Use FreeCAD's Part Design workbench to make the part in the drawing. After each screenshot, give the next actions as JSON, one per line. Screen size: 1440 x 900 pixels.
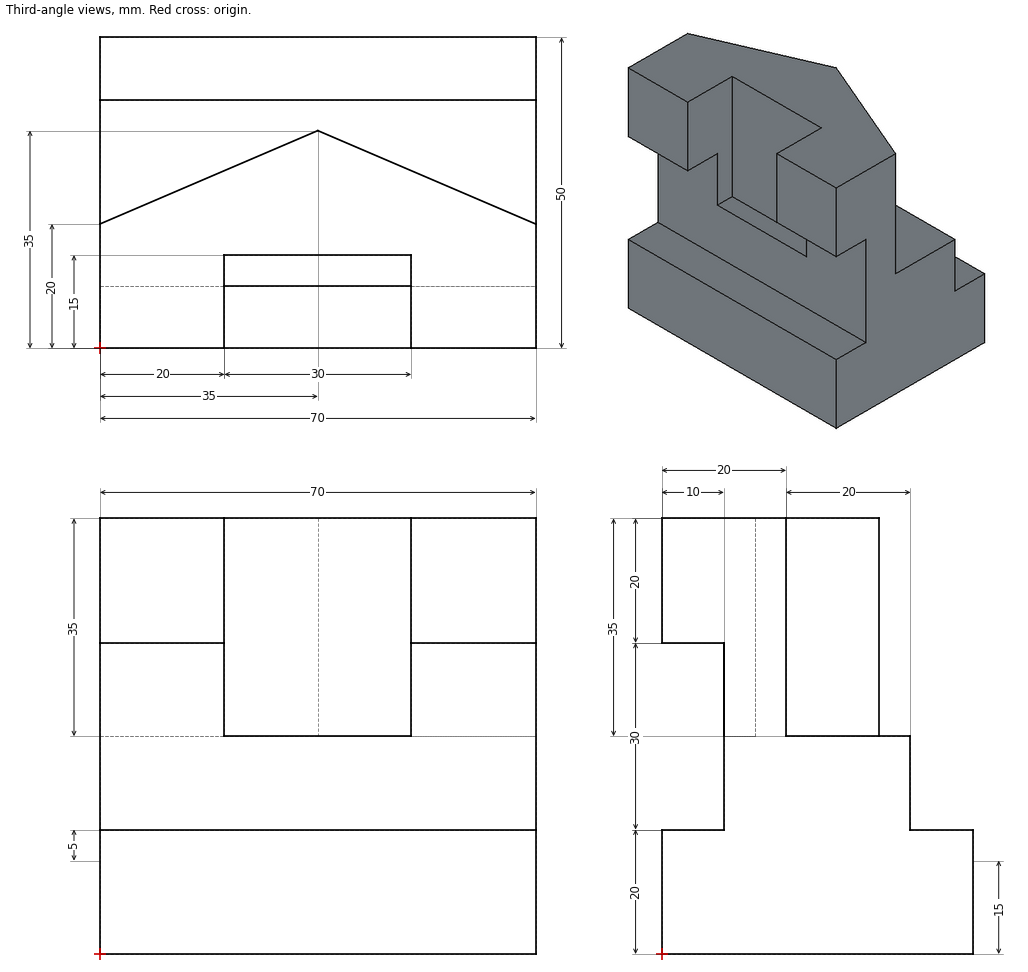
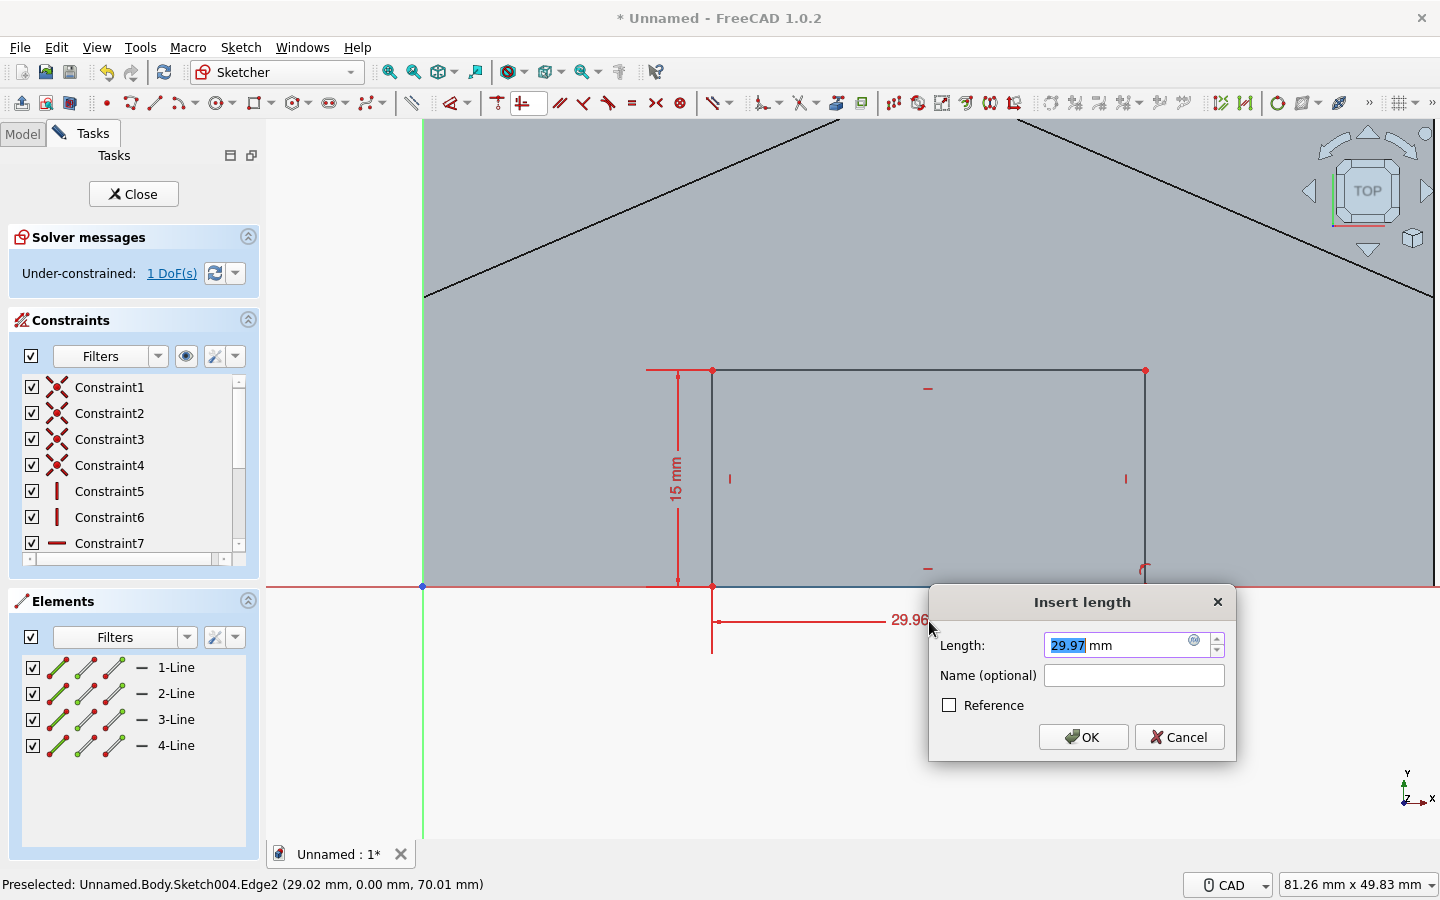
{"action": "type", "text": "30"}
{"action": "key", "text": "Return"}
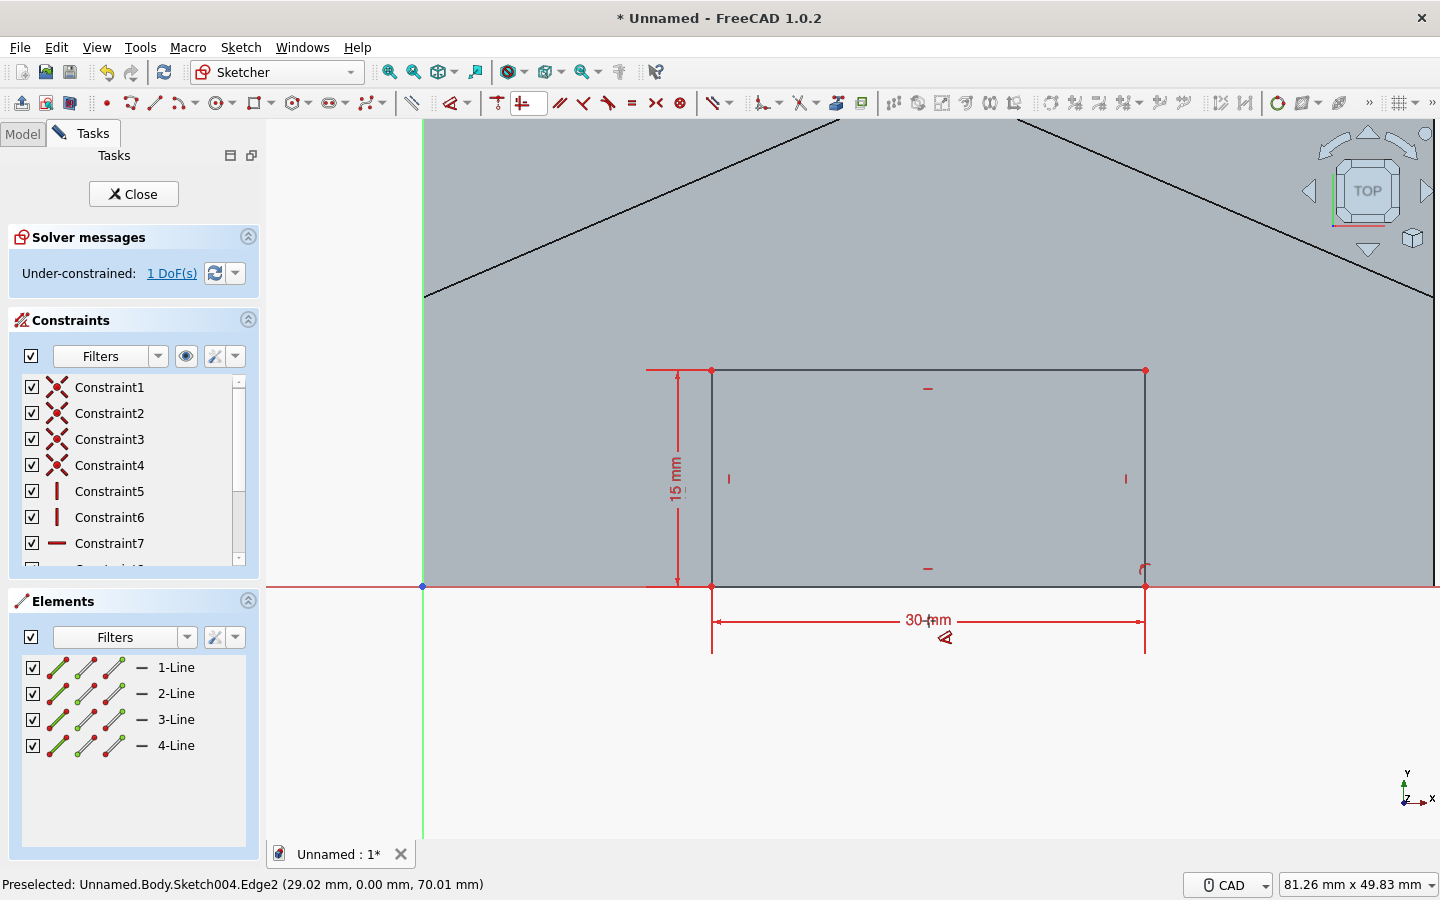
{"action": "left_click", "coordinate": [712, 370]}
{"action": "left_click", "coordinate": [567, 621]}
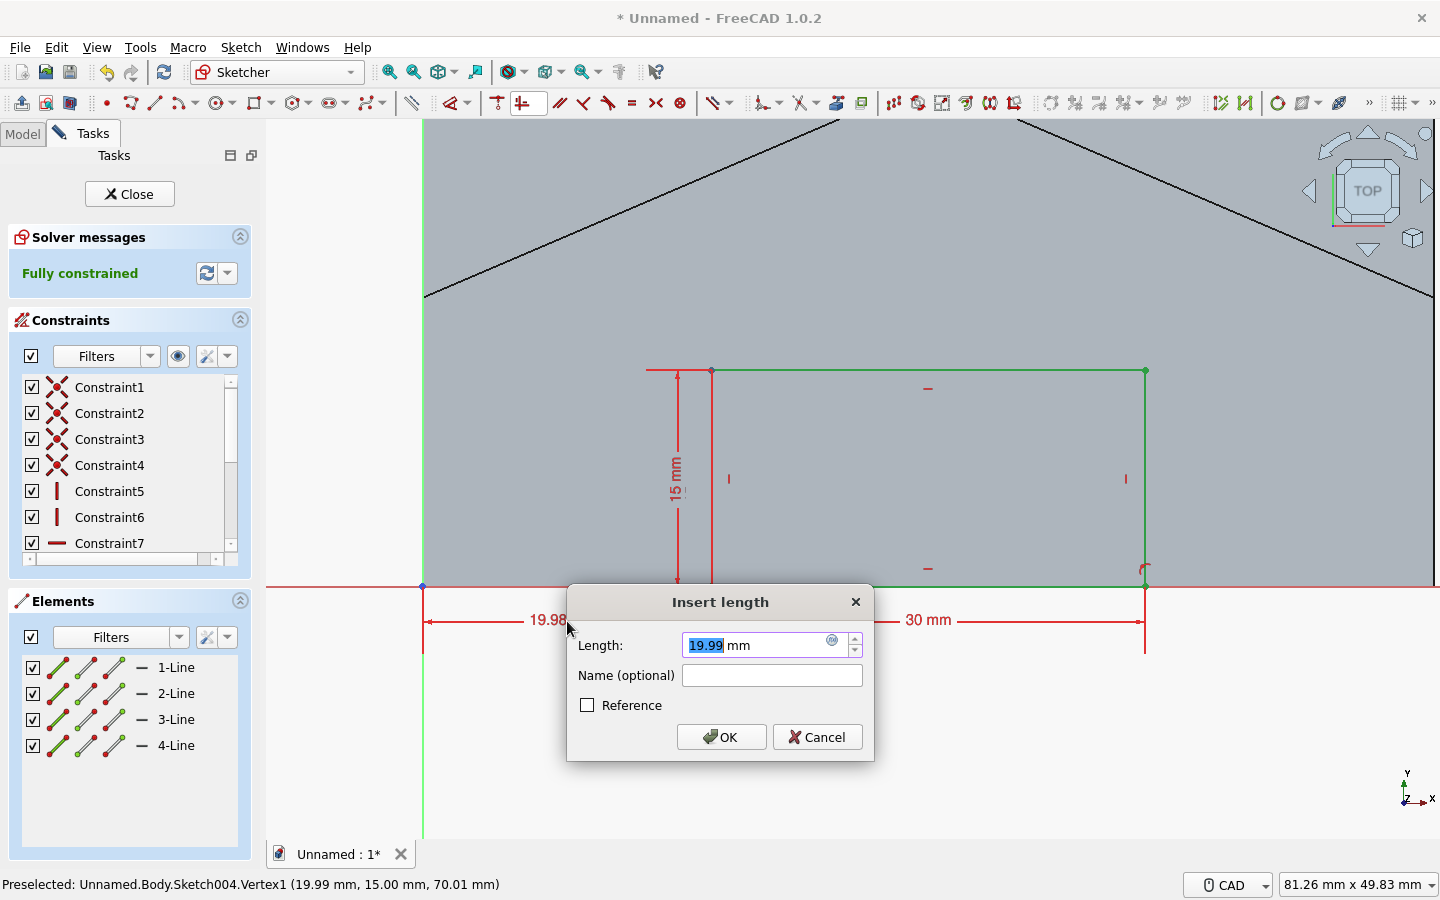
{"action": "type", "text": "20"}
{"action": "key", "text": "Return"}
{"action": "key", "text": "Escape"}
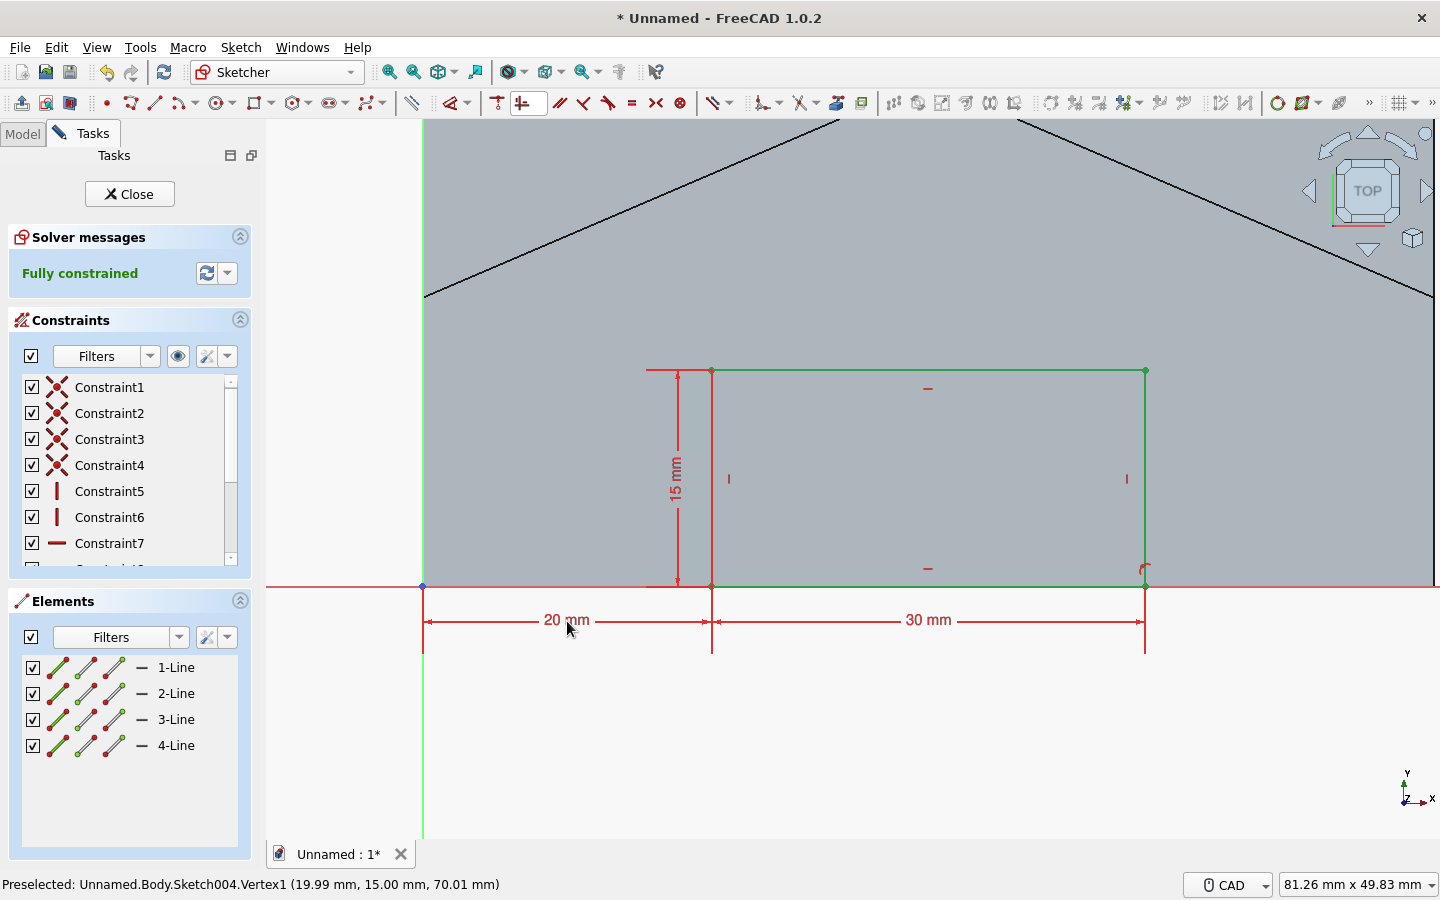
{"action": "left_click", "coordinate": [130, 194]}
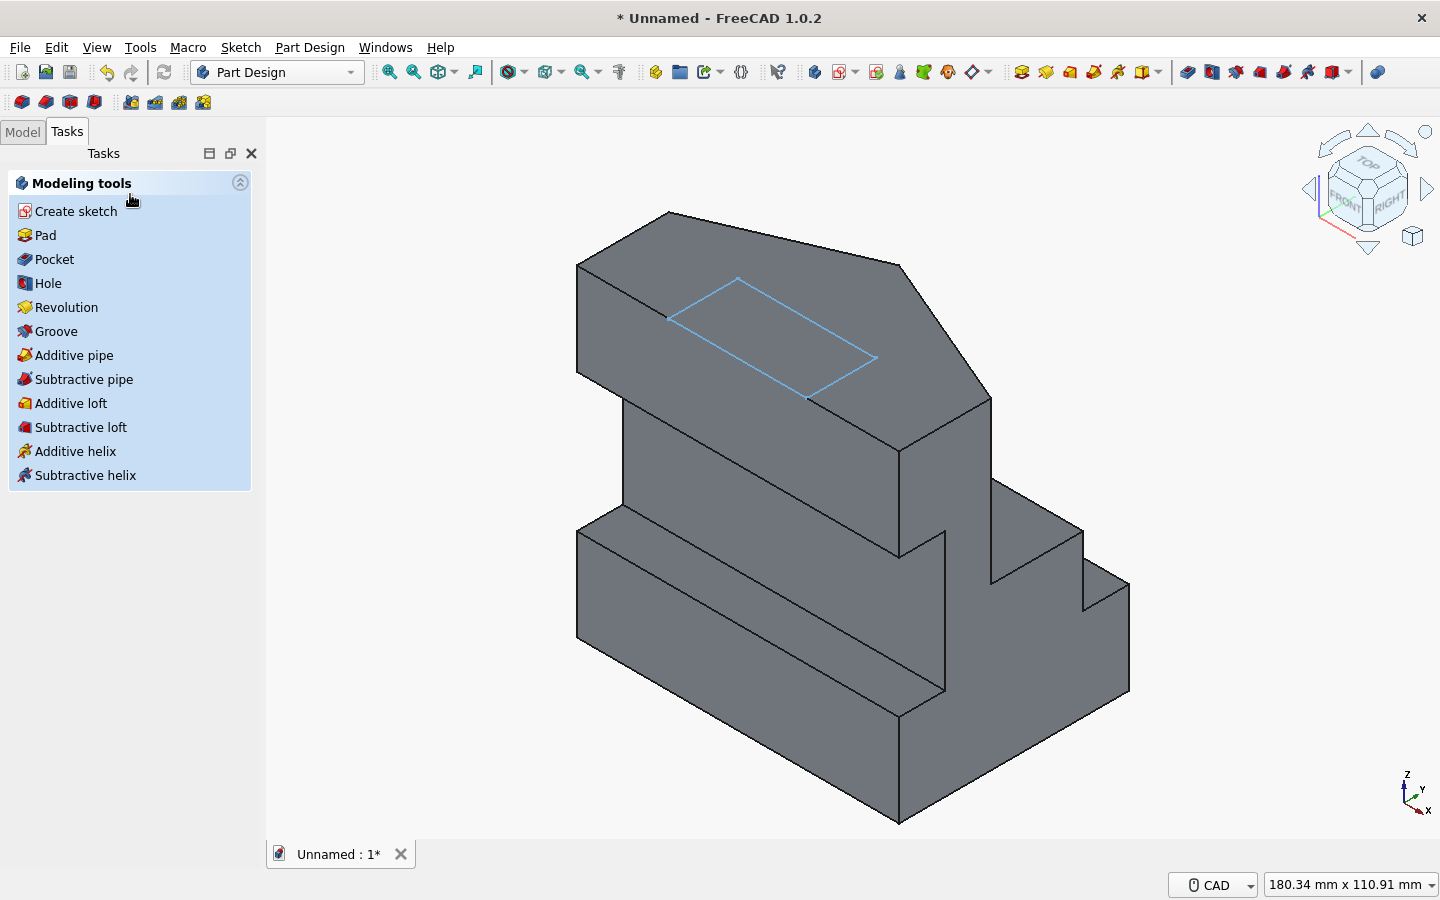
{"action": "left_click", "coordinate": [1188, 72]}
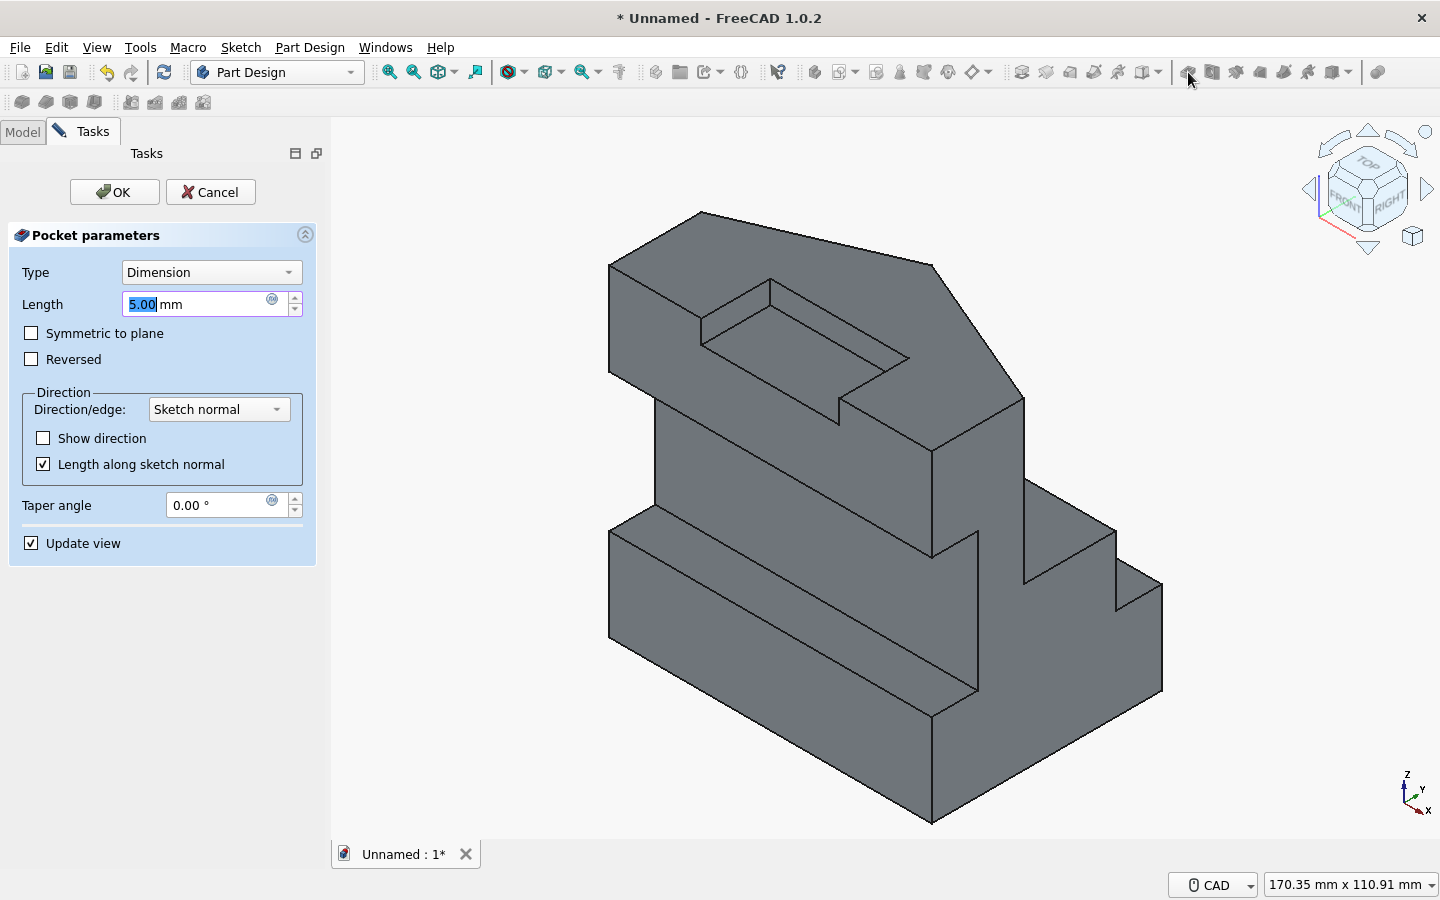
{"action": "type", "text": "35"}
{"action": "key", "text": "Tab"}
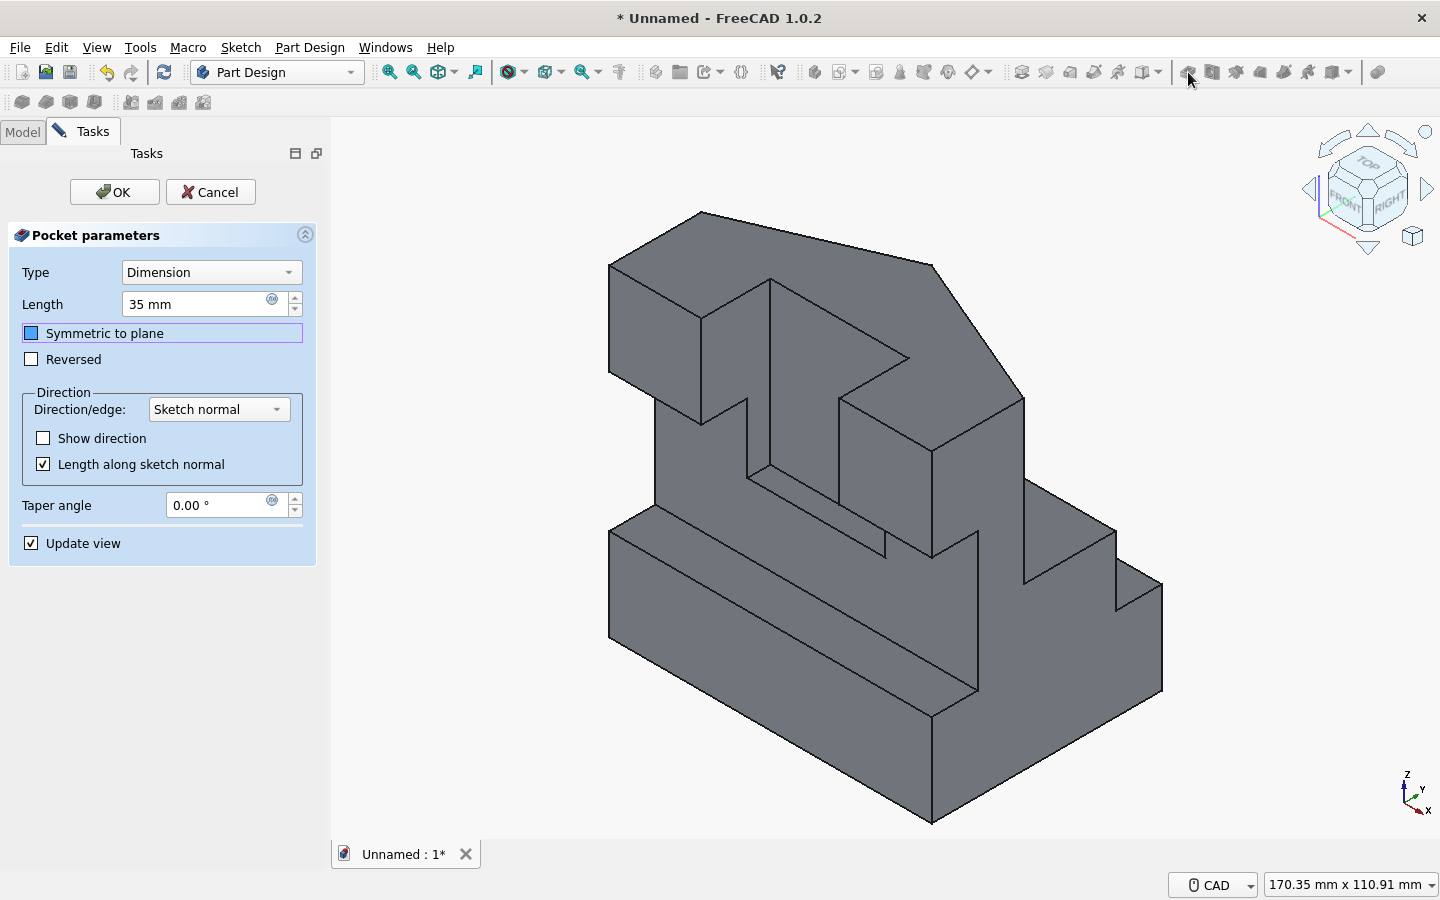
{"action": "left_click", "coordinate": [115, 192]}